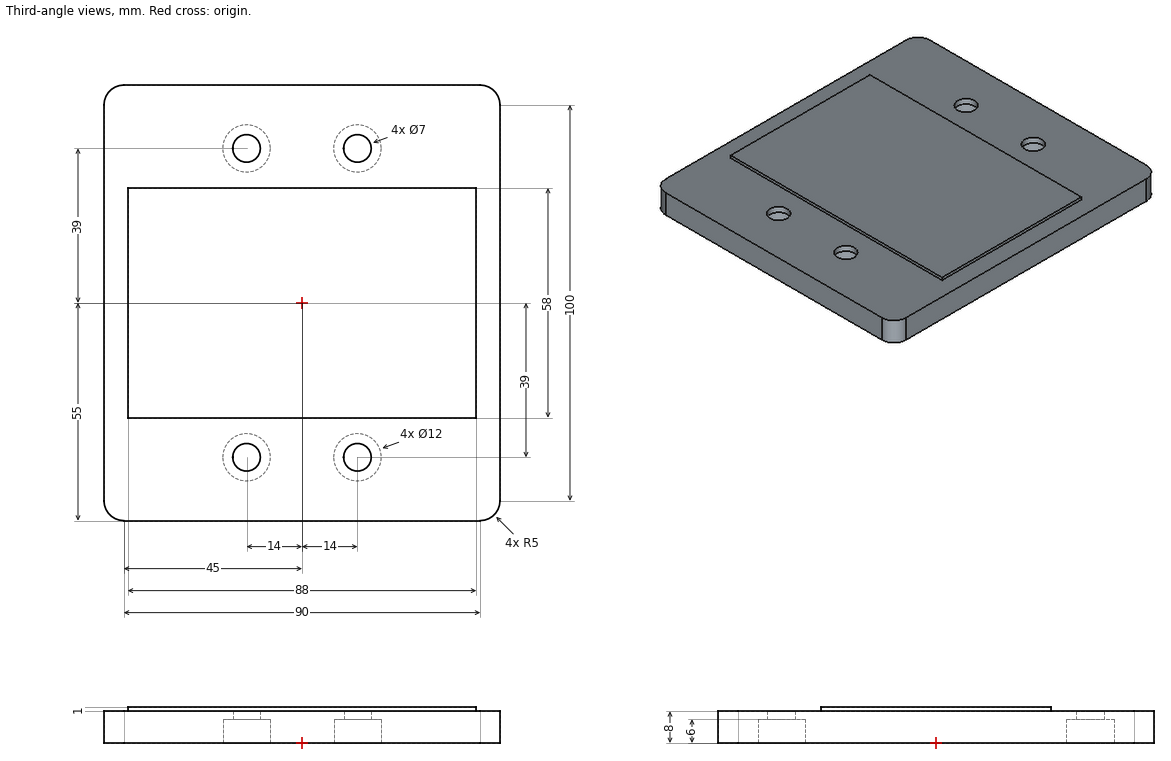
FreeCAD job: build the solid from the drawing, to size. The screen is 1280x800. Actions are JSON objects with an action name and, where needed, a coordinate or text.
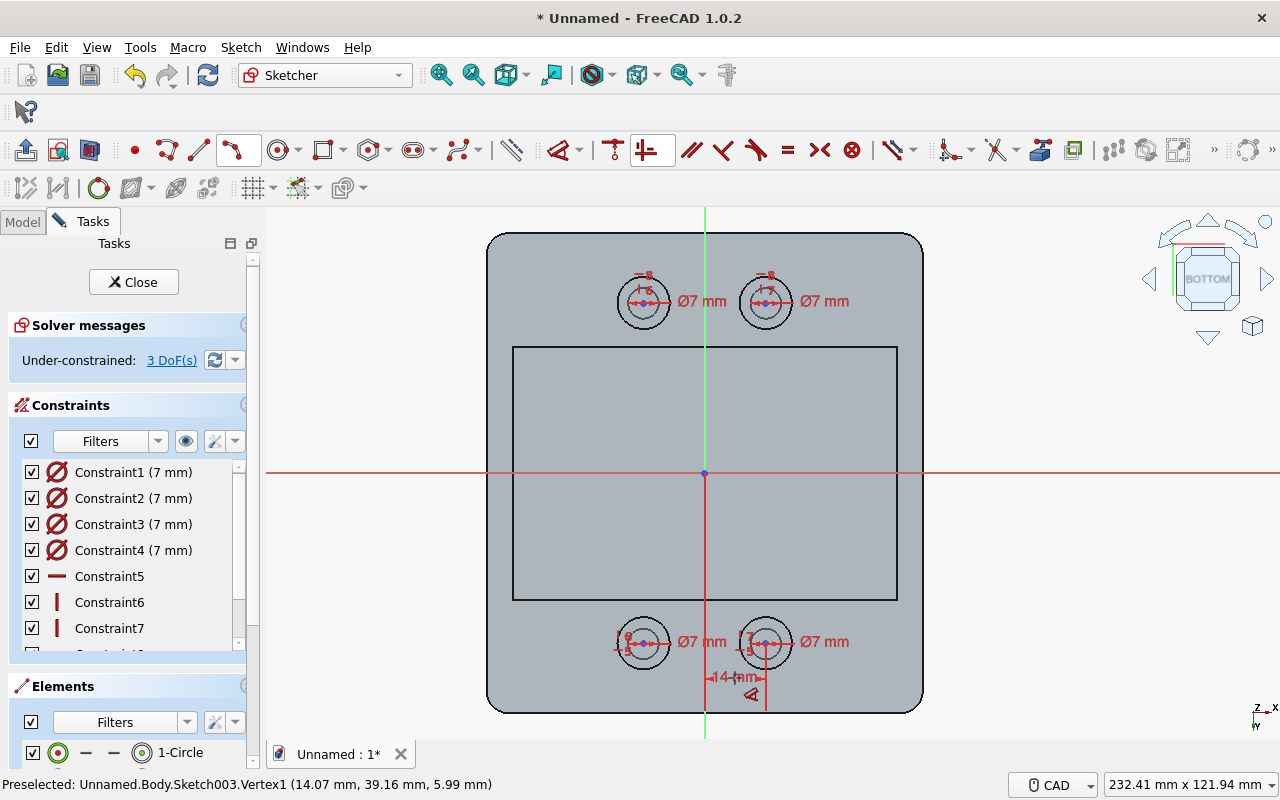
{"action": "left_click", "coordinate": [766, 644]}
{"action": "left_click", "coordinate": [800, 559]}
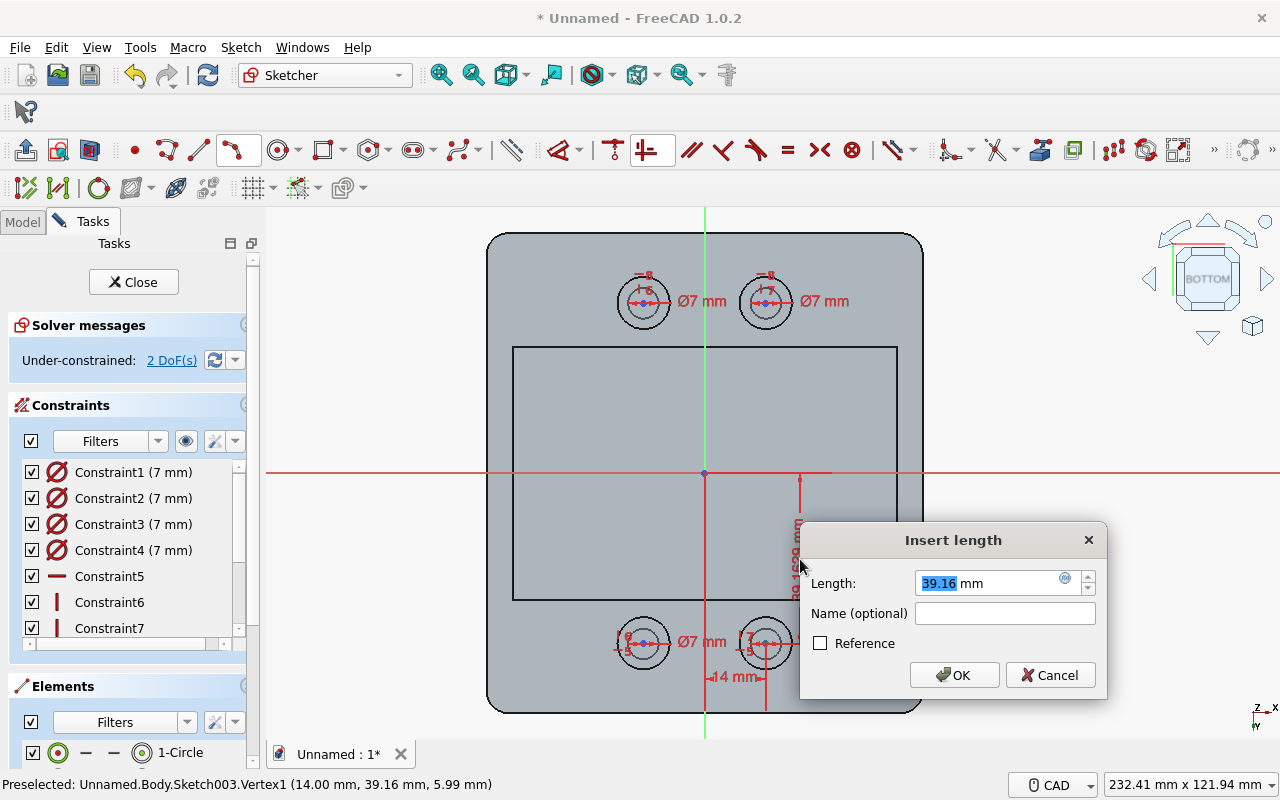
{"action": "type", "text": "39"}
{"action": "key", "text": "Return"}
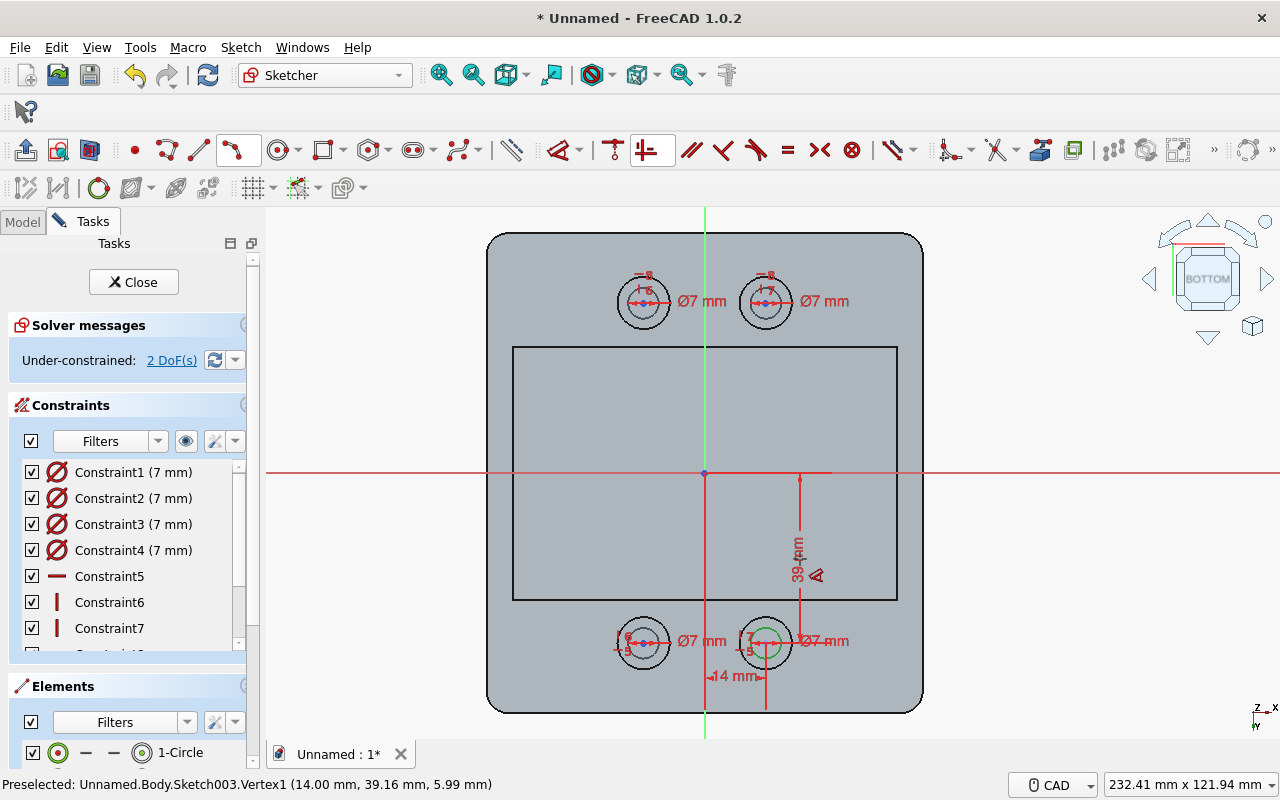
{"action": "left_click", "coordinate": [643, 643]}
{"action": "left_click", "coordinate": [660, 677]}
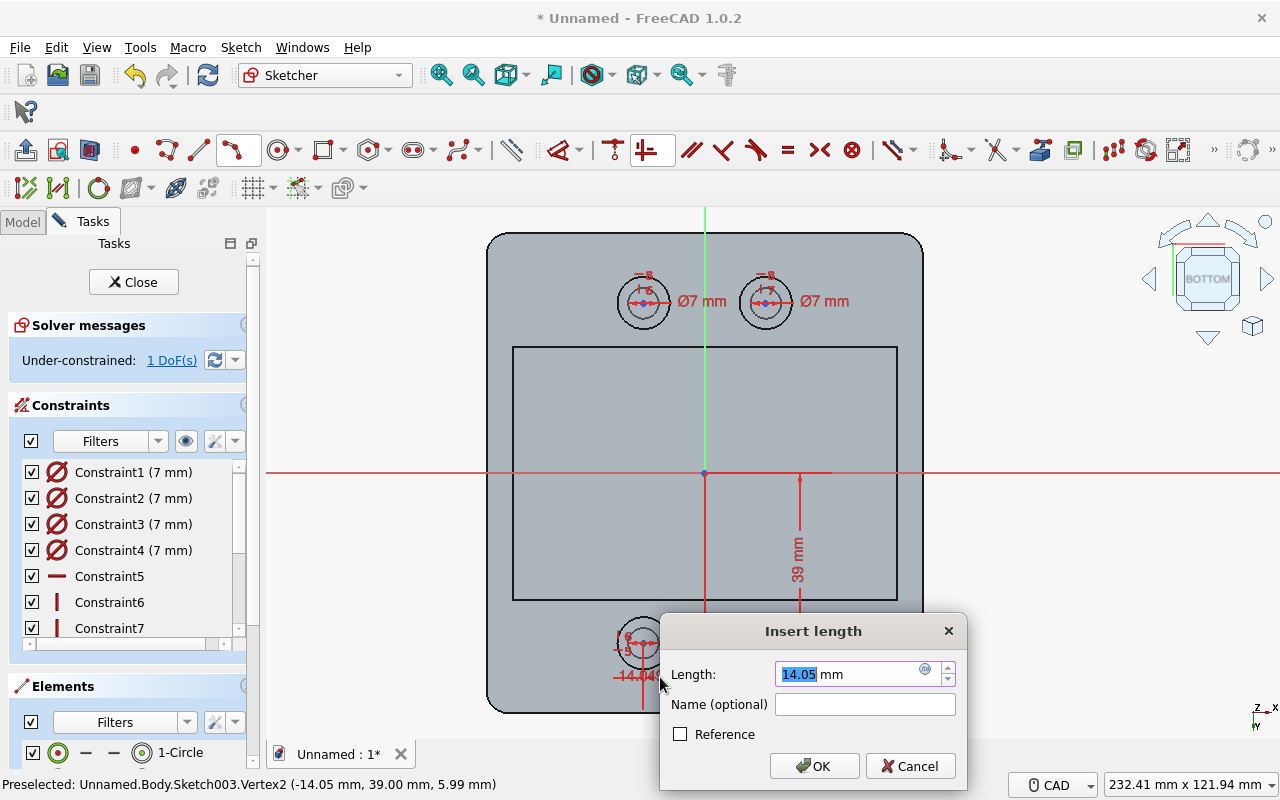
{"action": "type", "text": "14"}
{"action": "key", "text": "Return"}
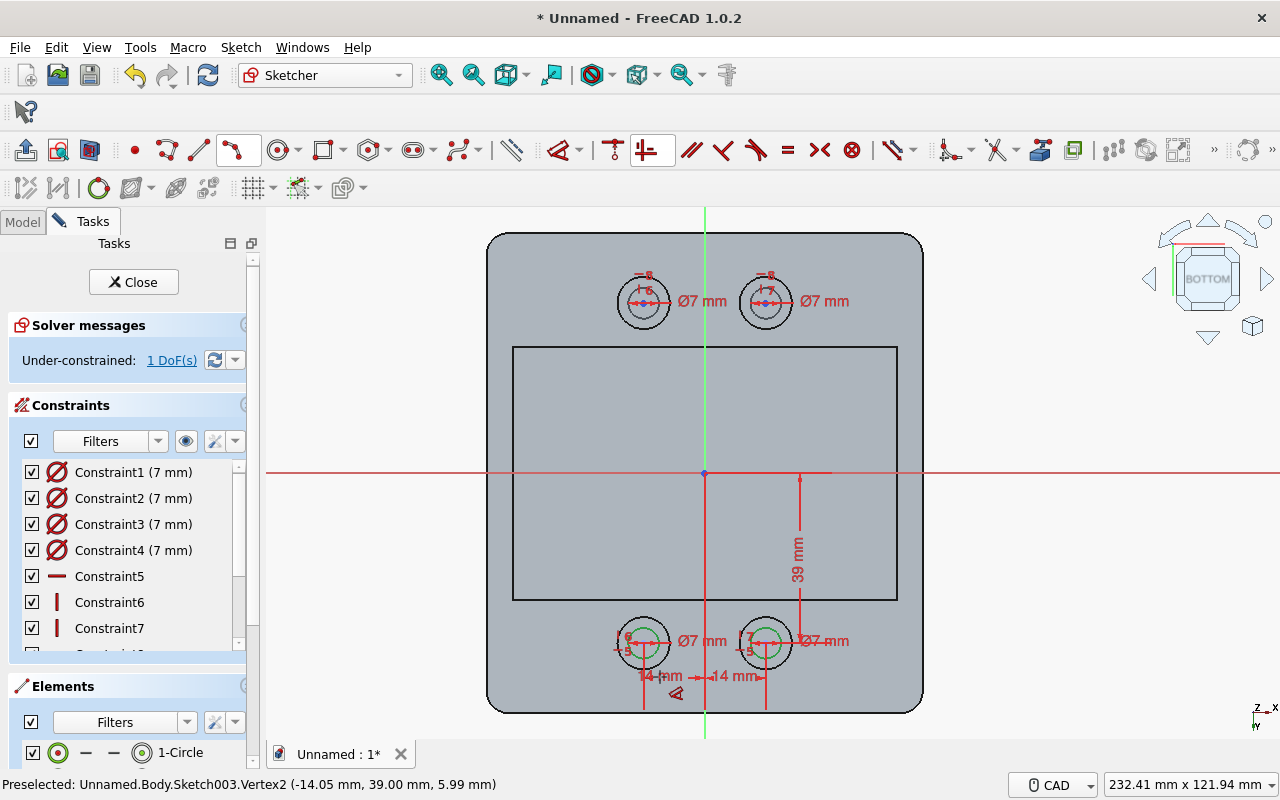
{"action": "left_click", "coordinate": [644, 303]}
{"action": "left_click", "coordinate": [610, 388]}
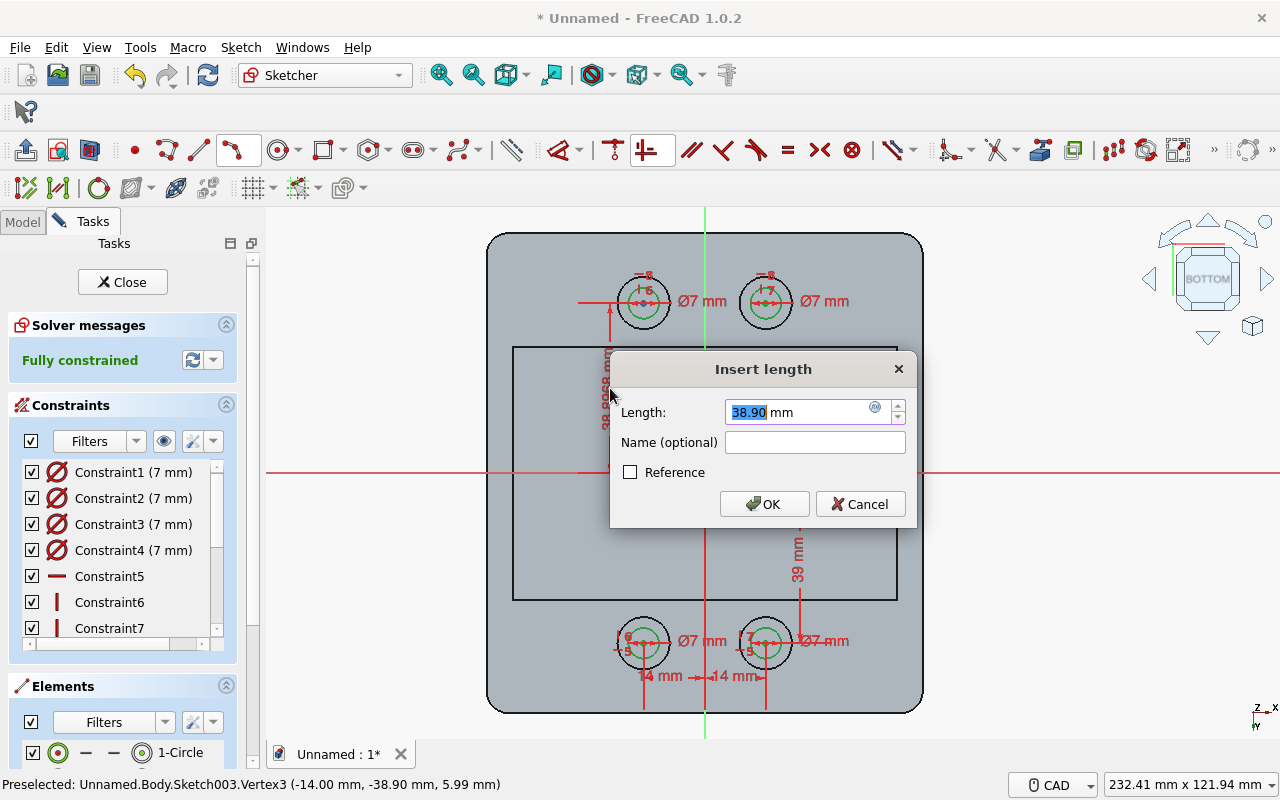
{"action": "type", "text": "39"}
{"action": "key", "text": "Return"}
{"action": "key", "text": "Escape"}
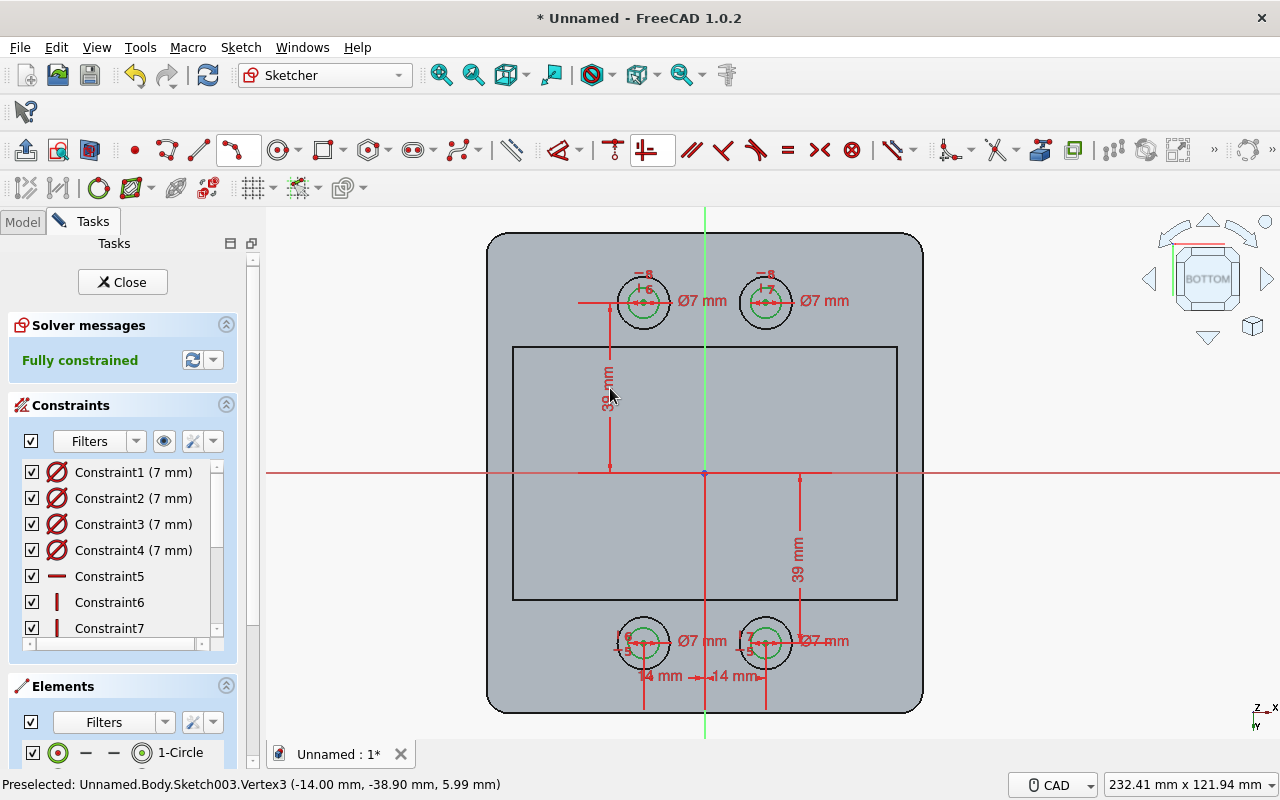
{"action": "left_click", "coordinate": [123, 282]}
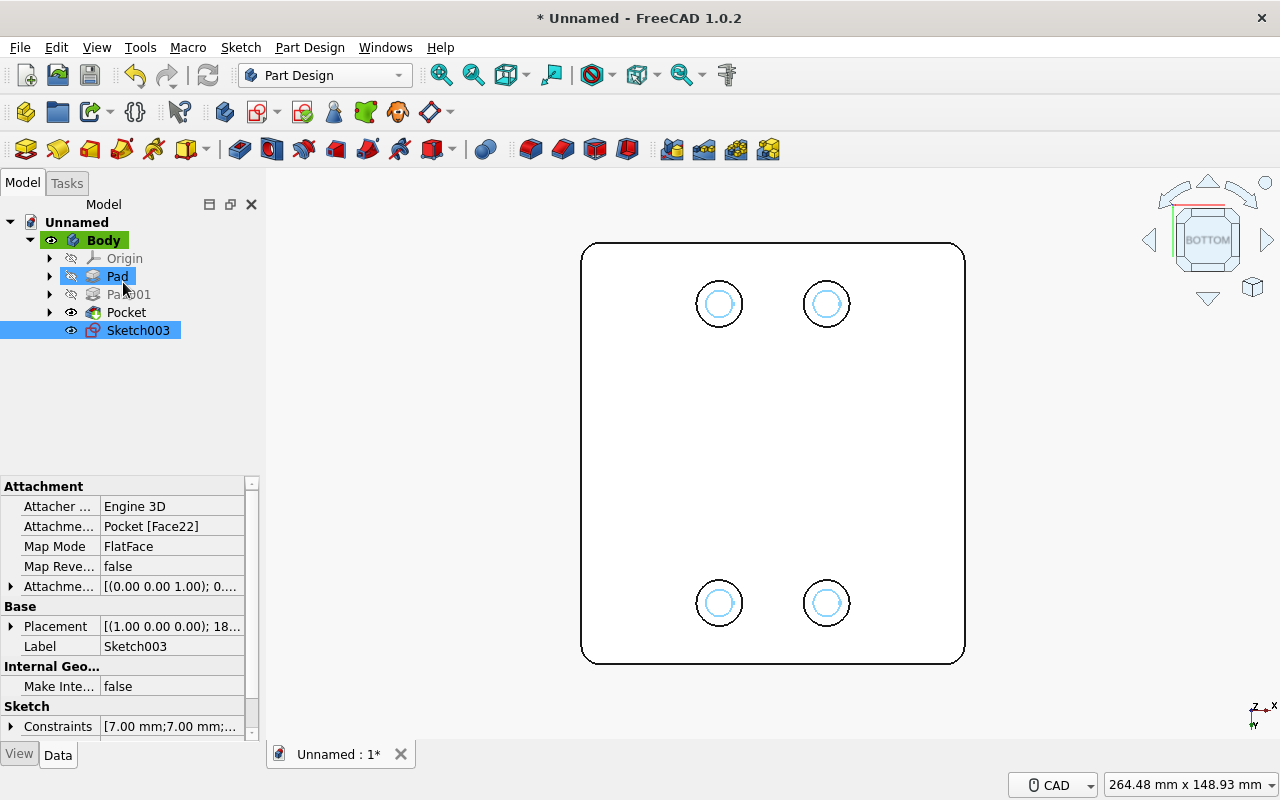
{"action": "left_click", "coordinate": [240, 150]}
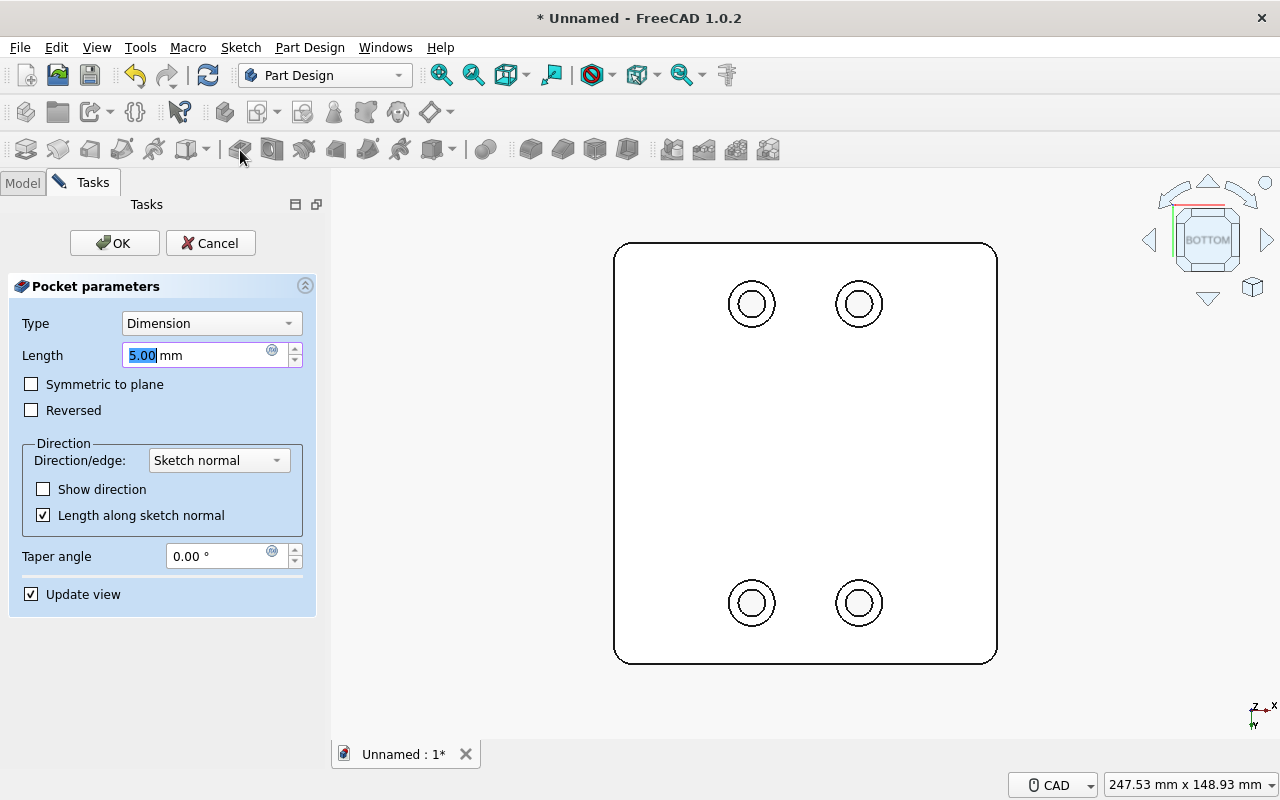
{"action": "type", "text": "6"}
{"action": "key", "text": "Tab"}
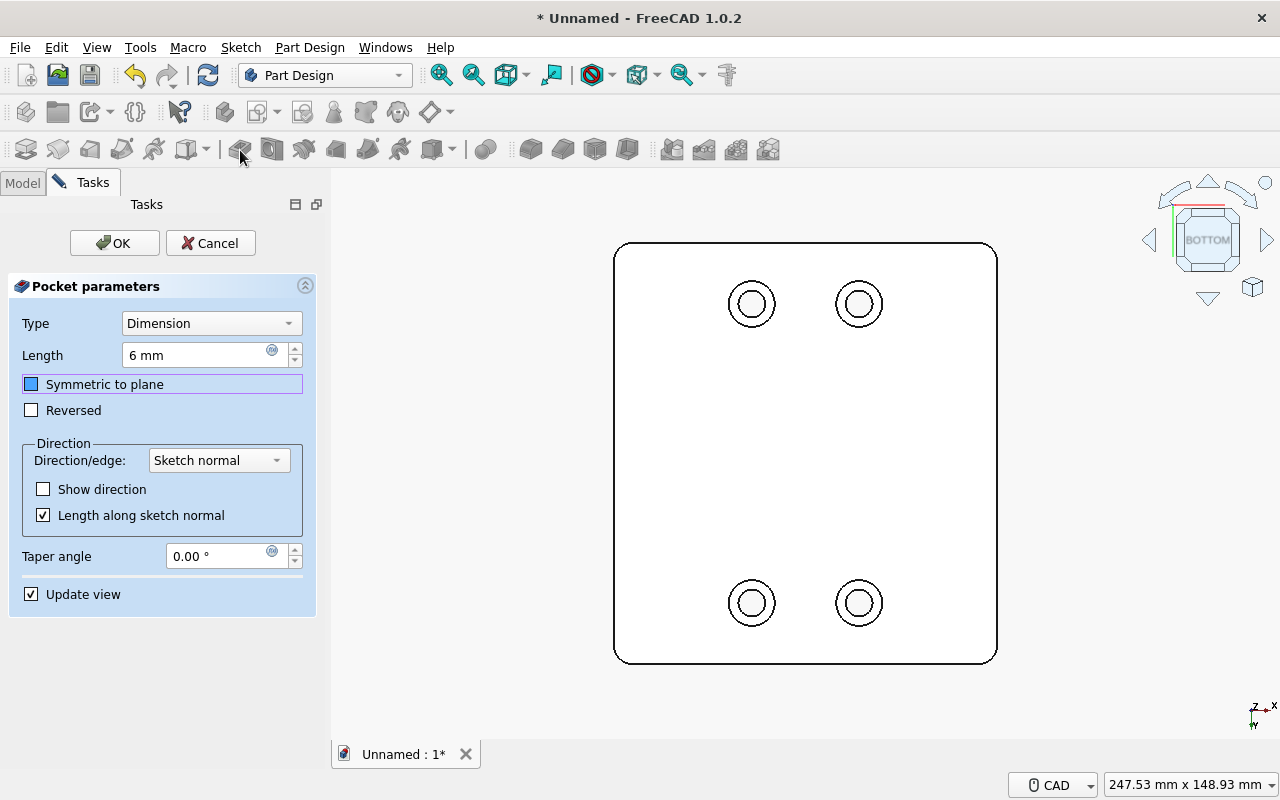
{"action": "left_click", "coordinate": [115, 243]}